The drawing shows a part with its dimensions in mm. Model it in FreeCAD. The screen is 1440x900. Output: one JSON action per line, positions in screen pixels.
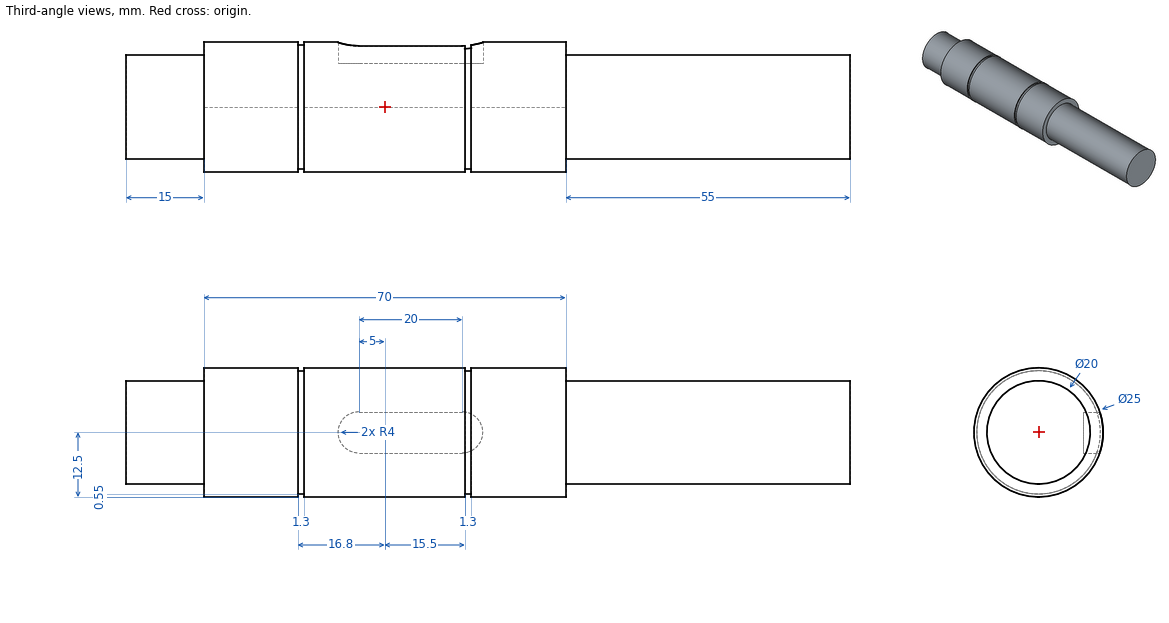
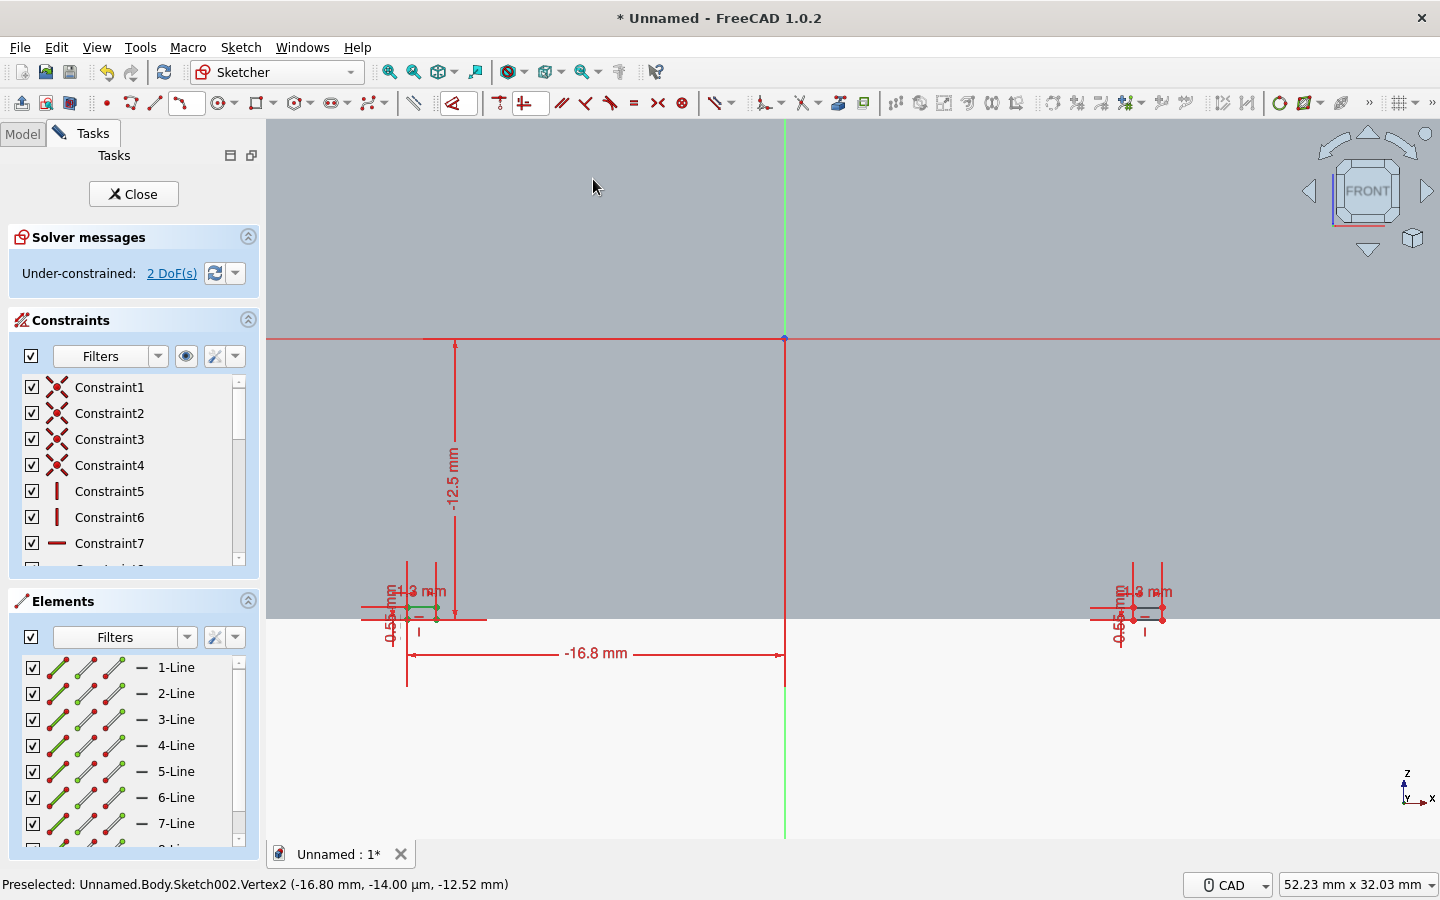
{"action": "left_click", "coordinate": [1133, 608]}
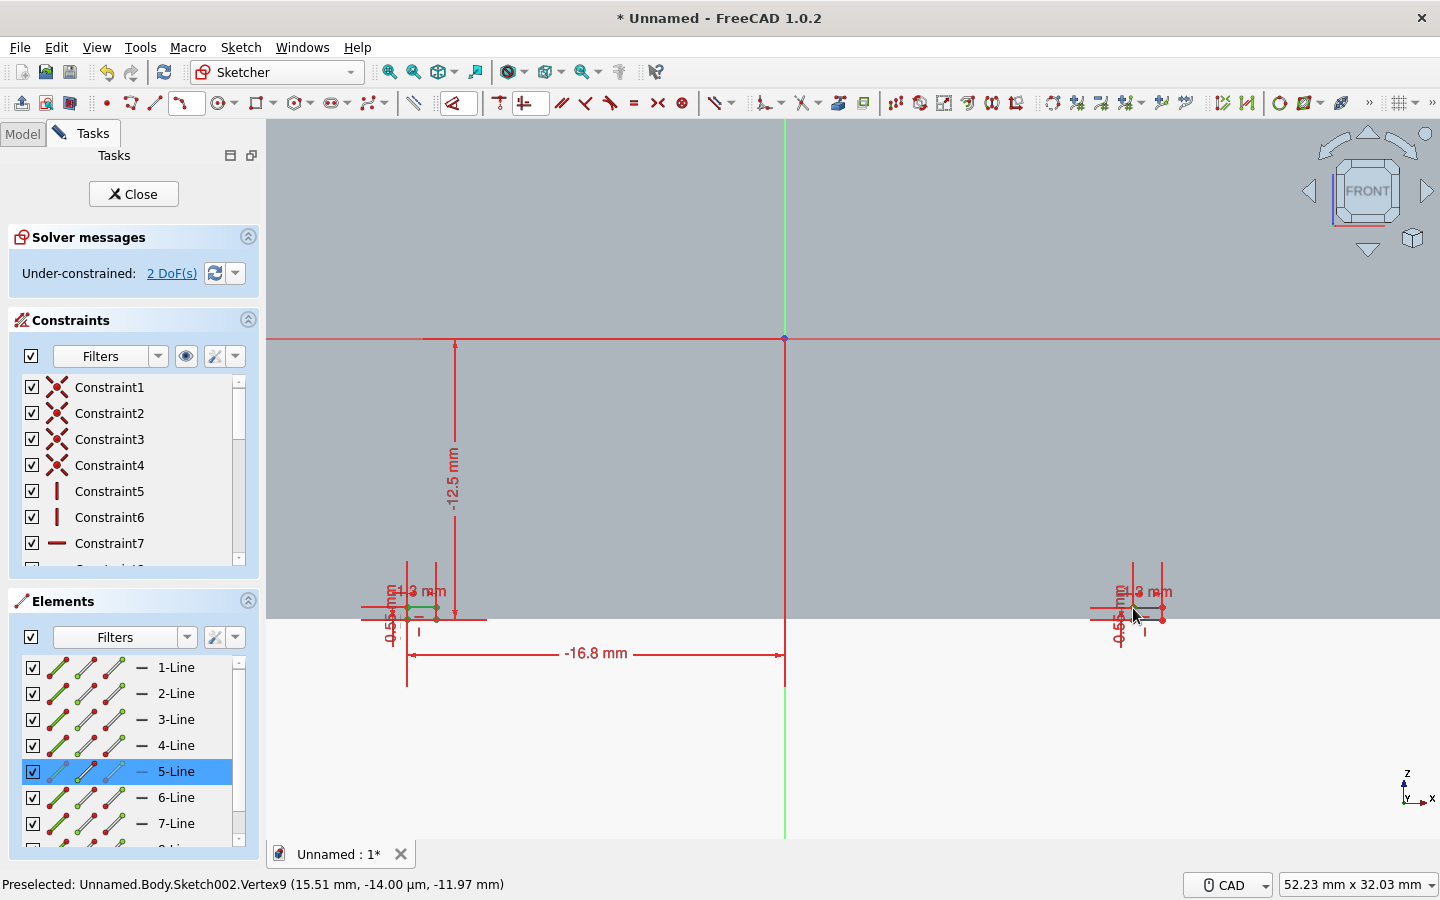
{"action": "left_click", "coordinate": [472, 104]}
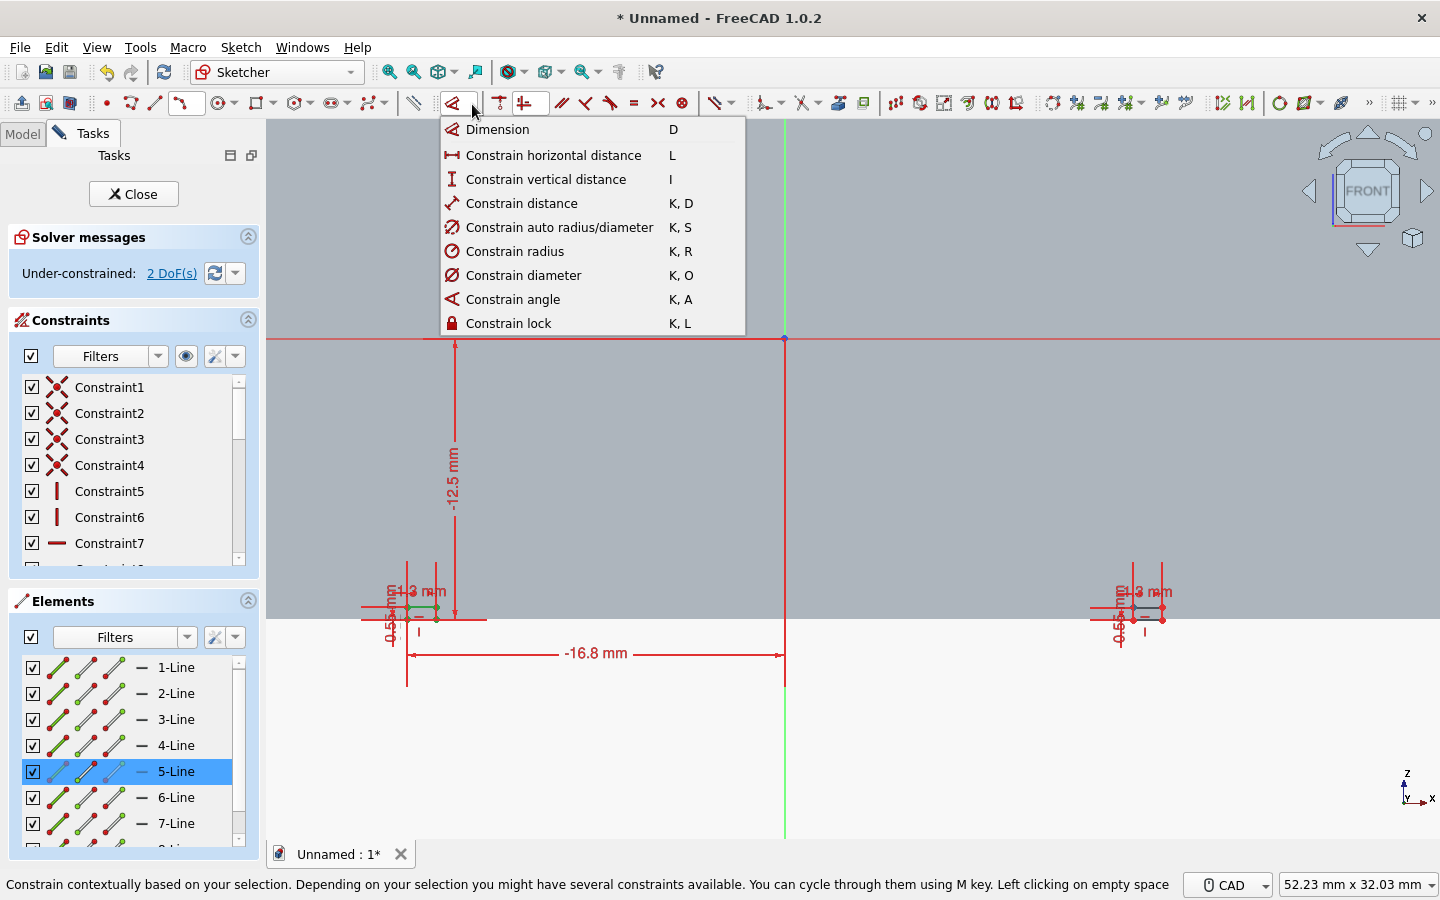
{"action": "left_click", "coordinate": [593, 155]}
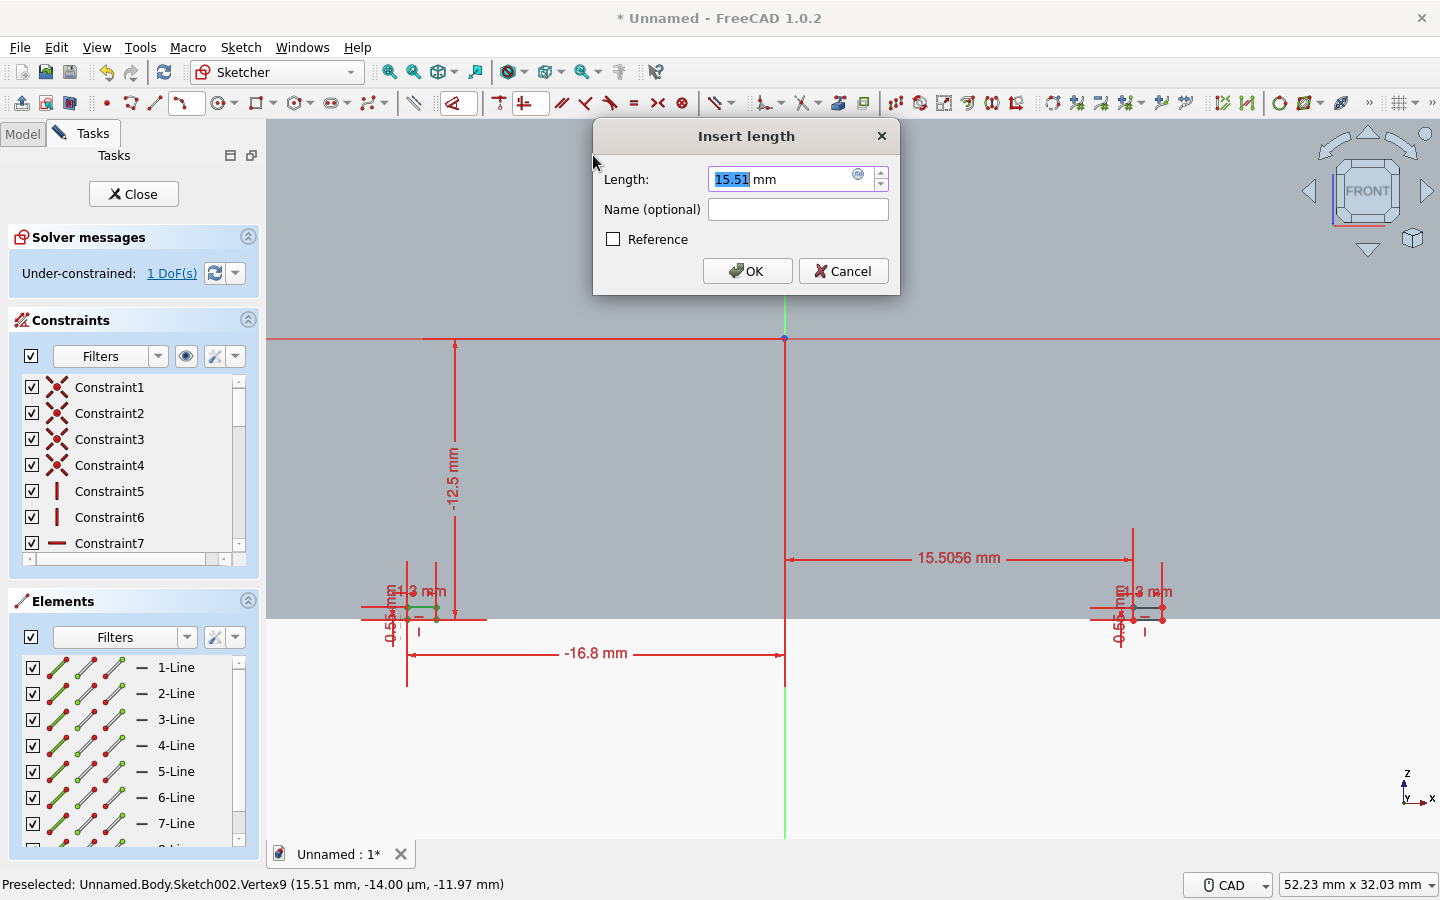
{"action": "type", "text": "15.5"}
{"action": "key", "text": "Return"}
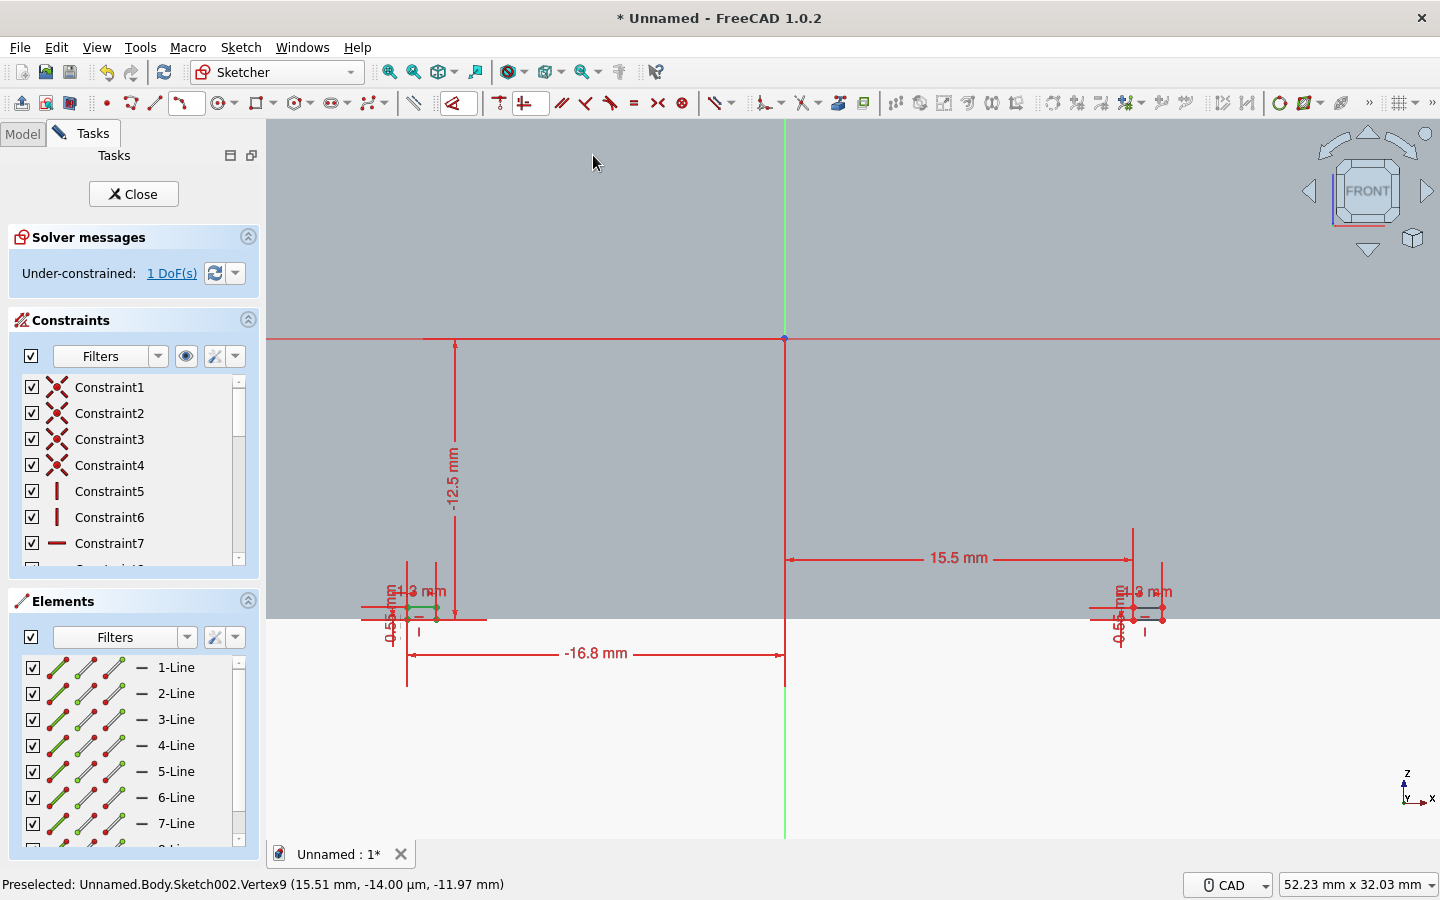
{"action": "left_click", "coordinate": [1133, 620]}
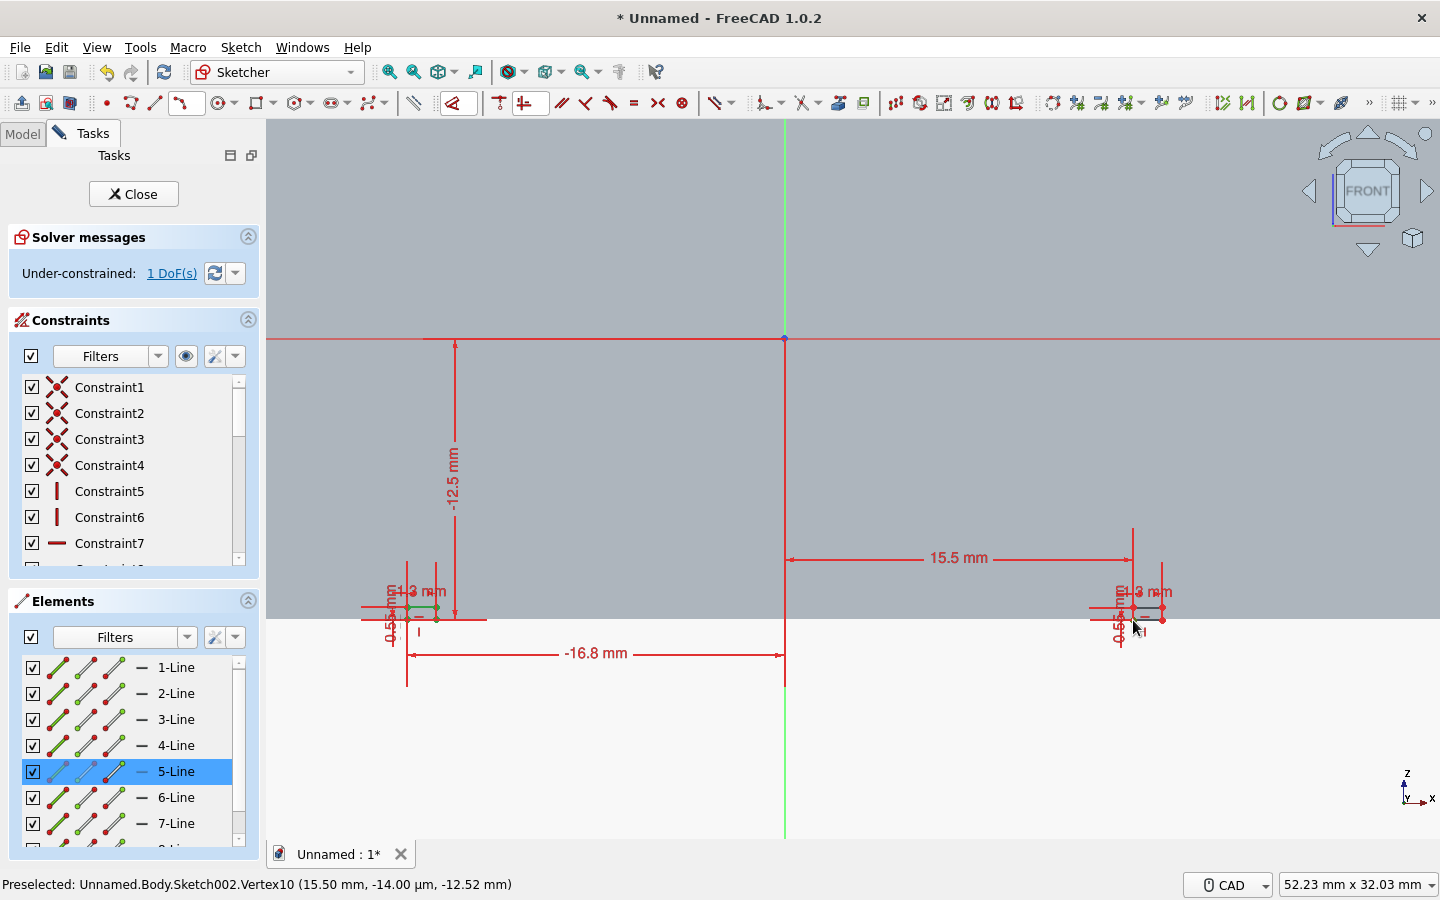
{"action": "key", "text": "i"}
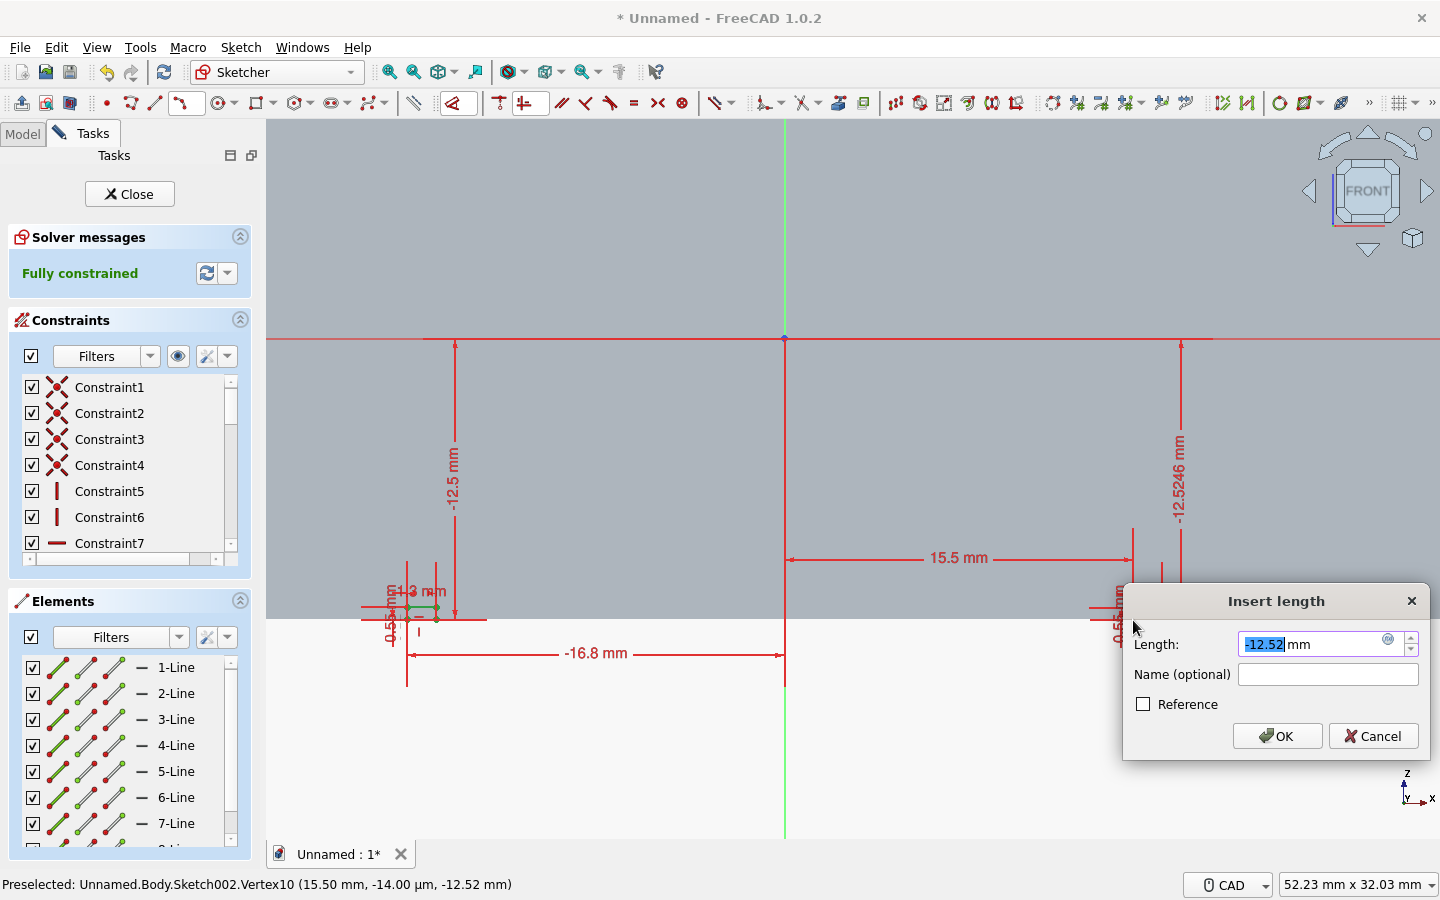
{"action": "type", "text": "-12.5"}
{"action": "key", "text": "Return"}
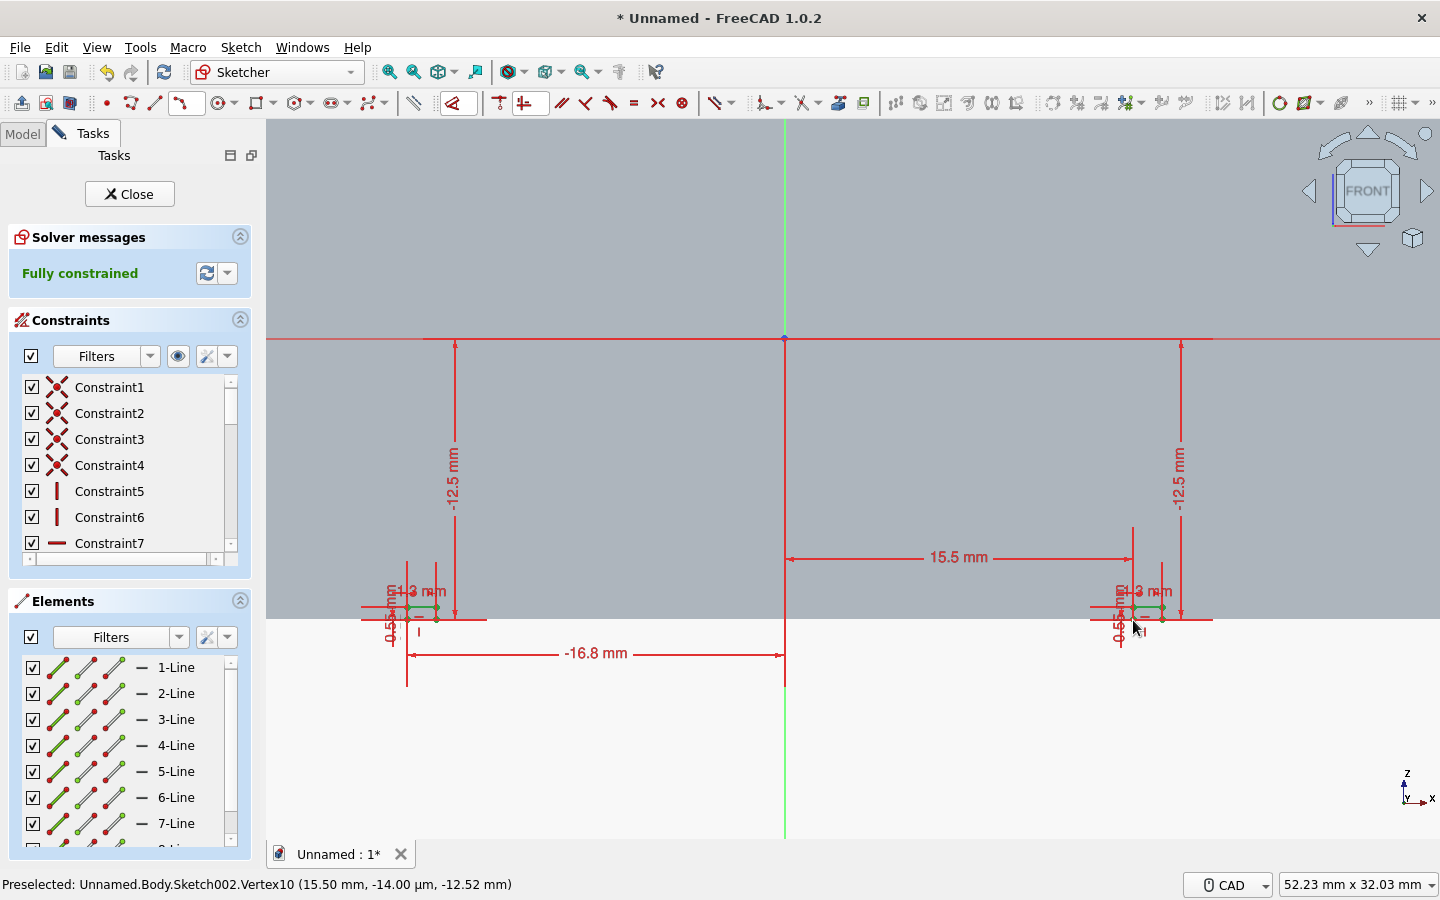
{"action": "left_click", "coordinate": [130, 194]}